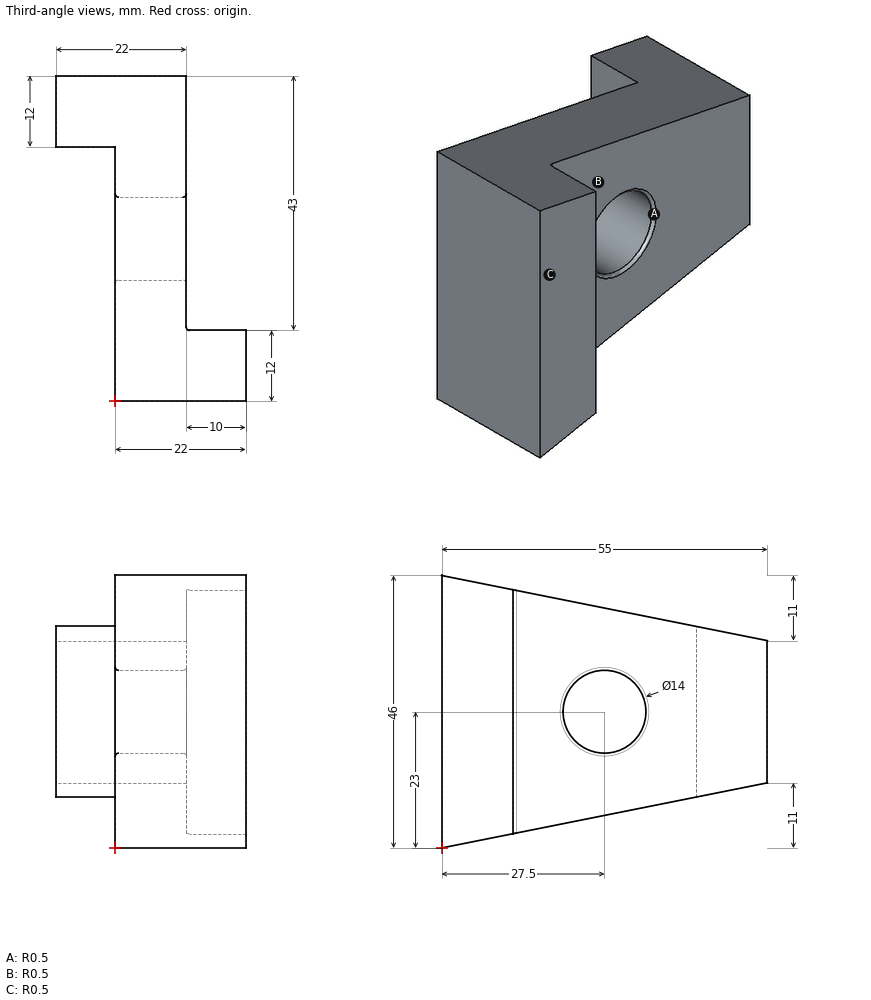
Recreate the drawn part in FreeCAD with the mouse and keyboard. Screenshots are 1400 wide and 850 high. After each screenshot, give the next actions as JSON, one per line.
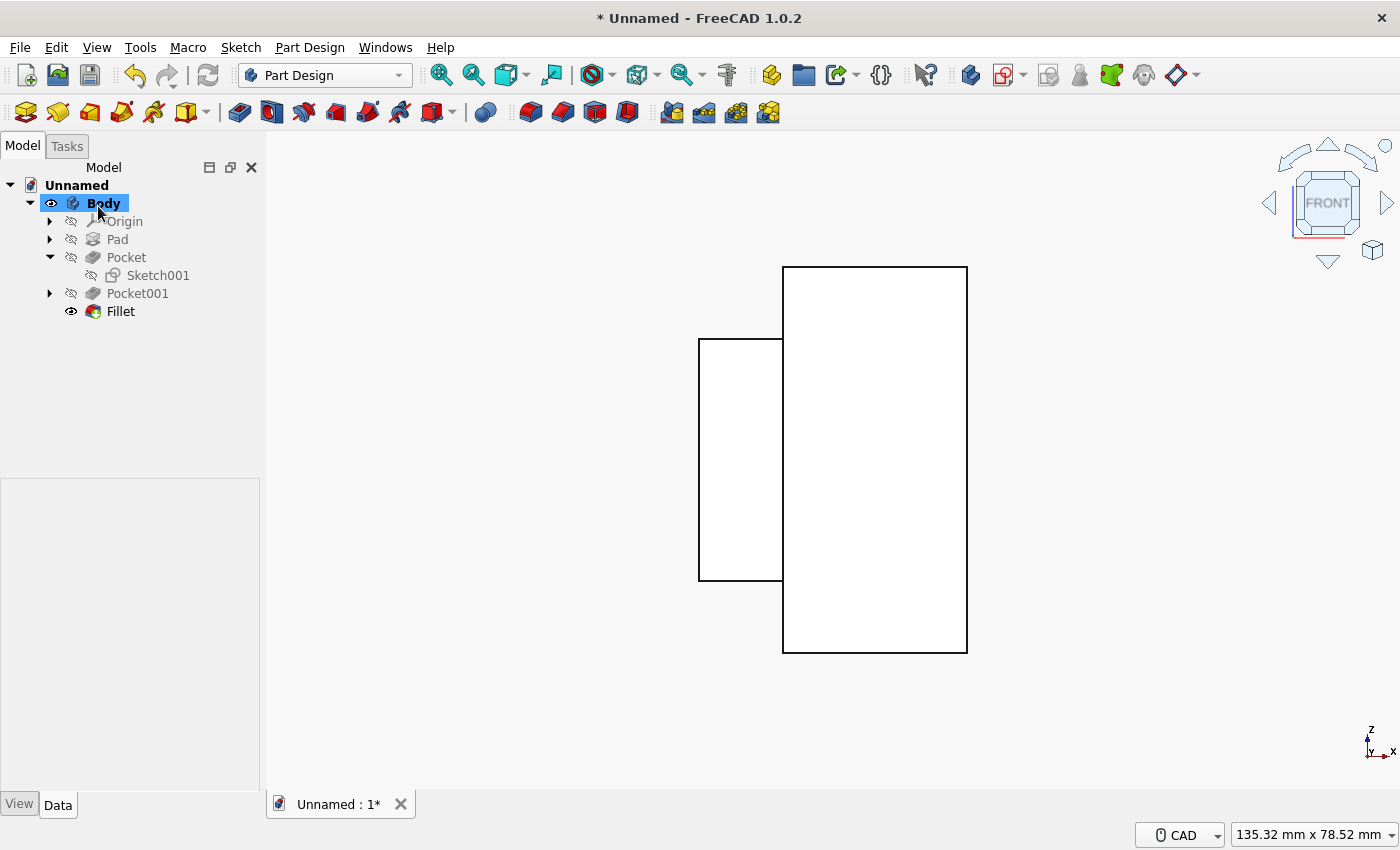
{"action": "key", "text": "3"}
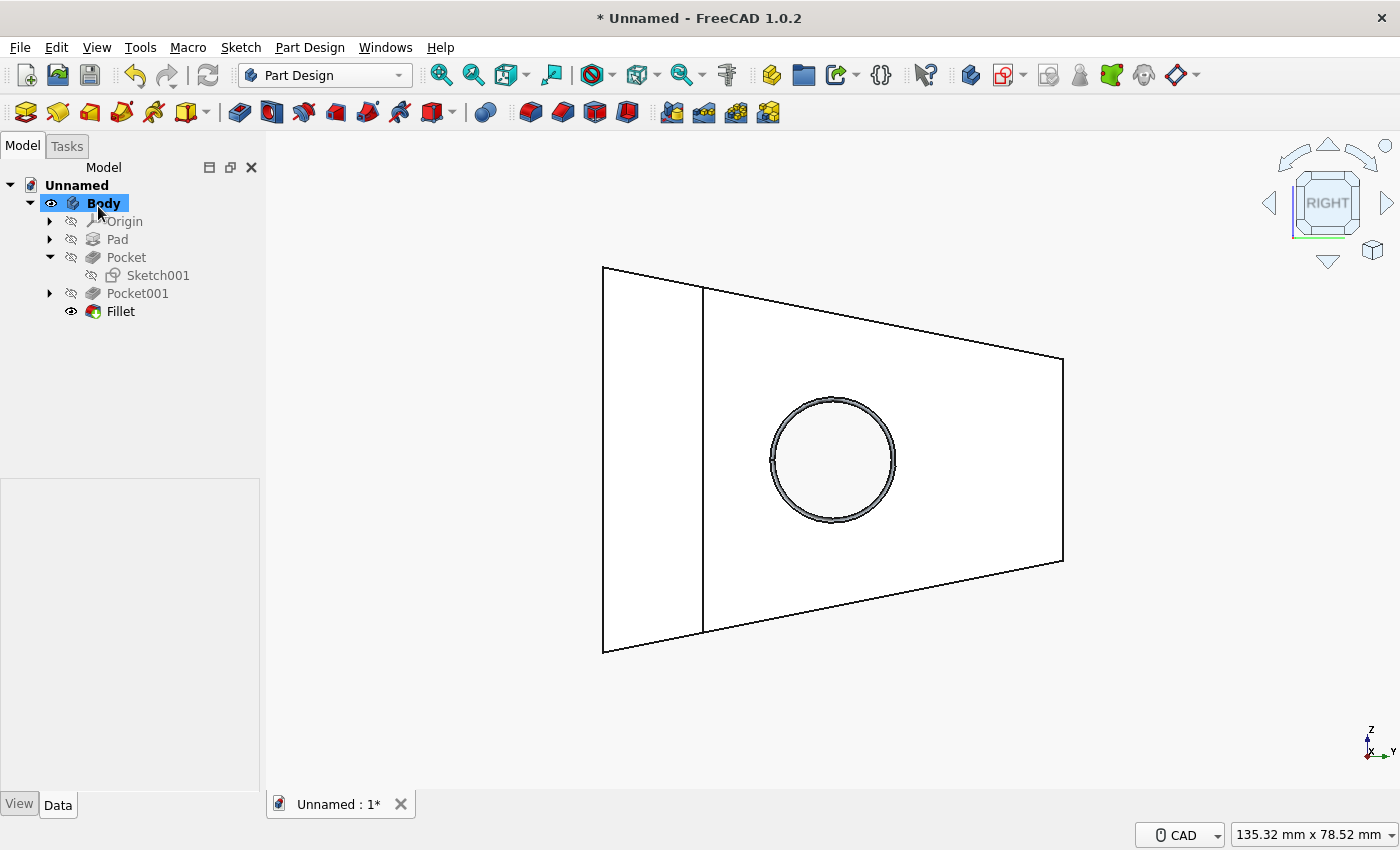
{"action": "key", "text": "5"}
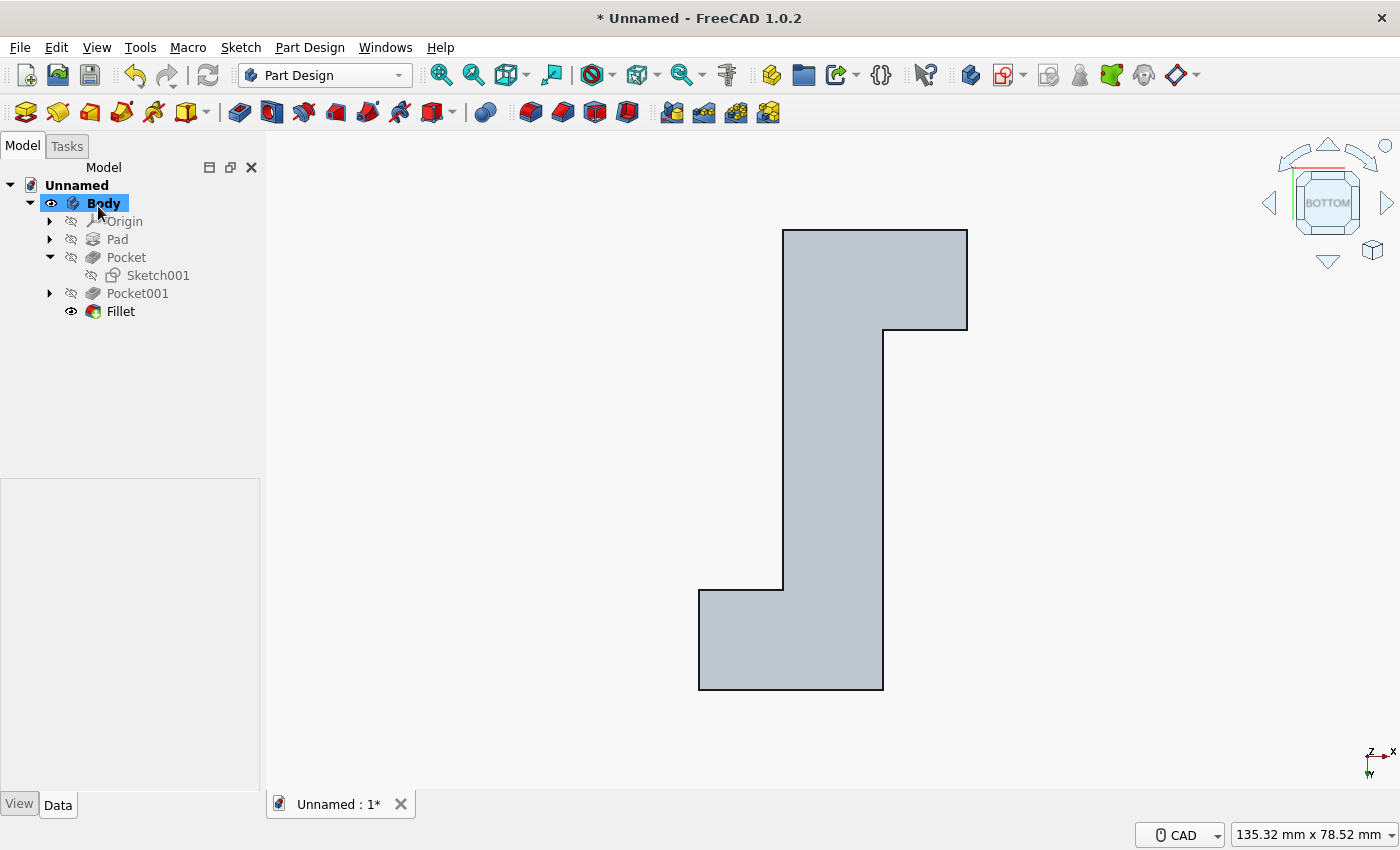
{"action": "key", "text": "4"}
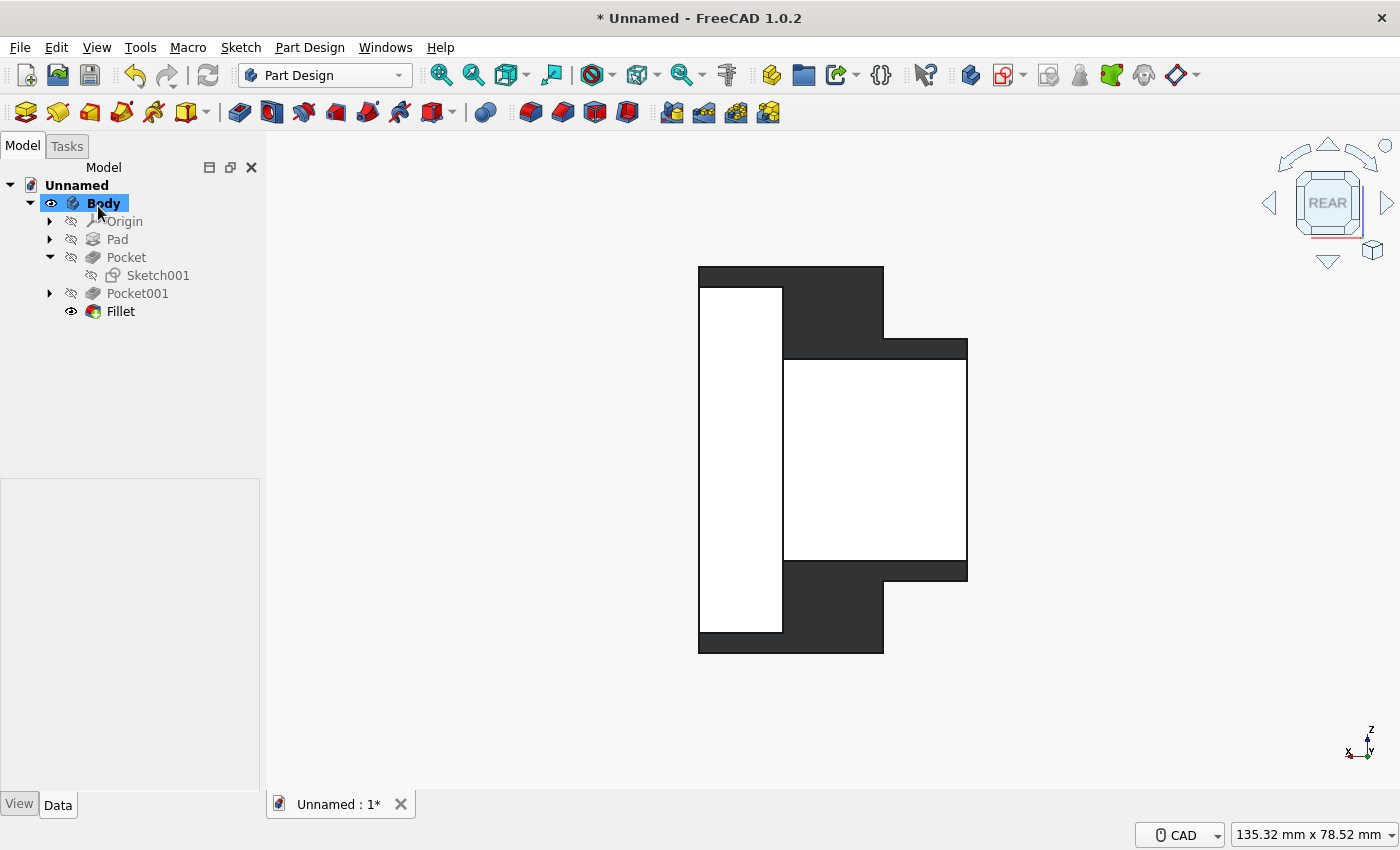
{"action": "key", "text": "6"}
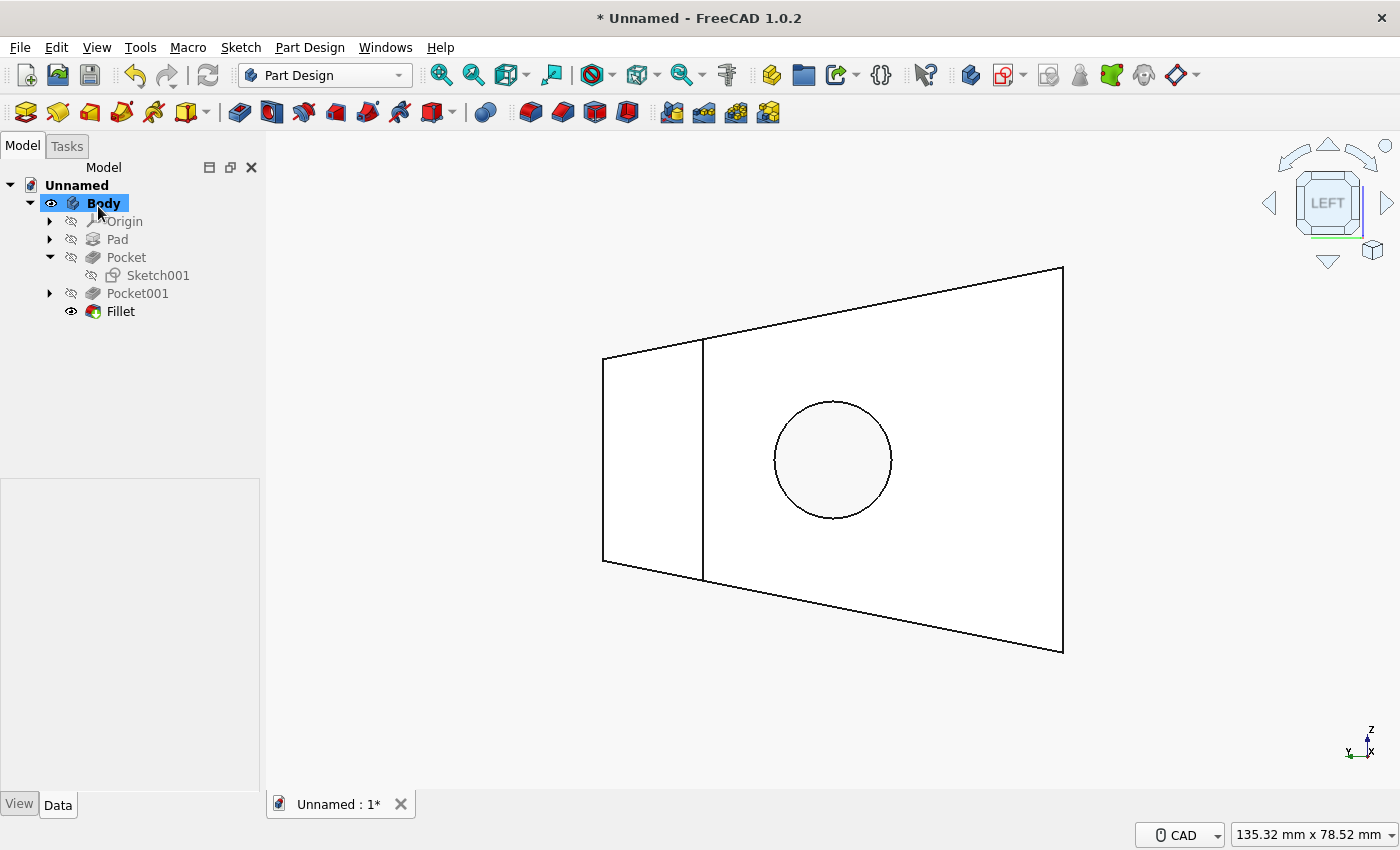
{"action": "left_click", "coordinate": [774, 459]}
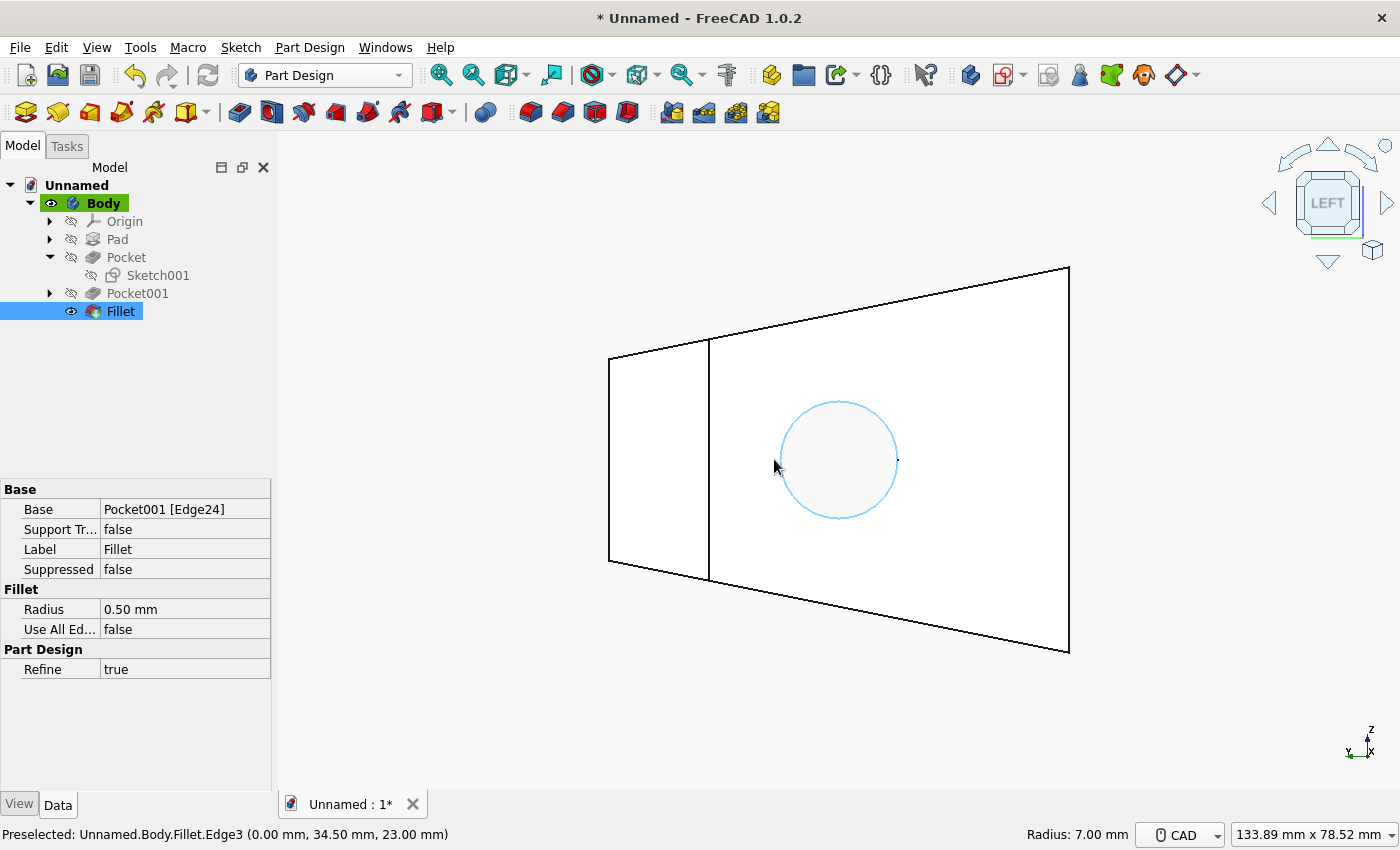
{"action": "left_click", "coordinate": [532, 112]}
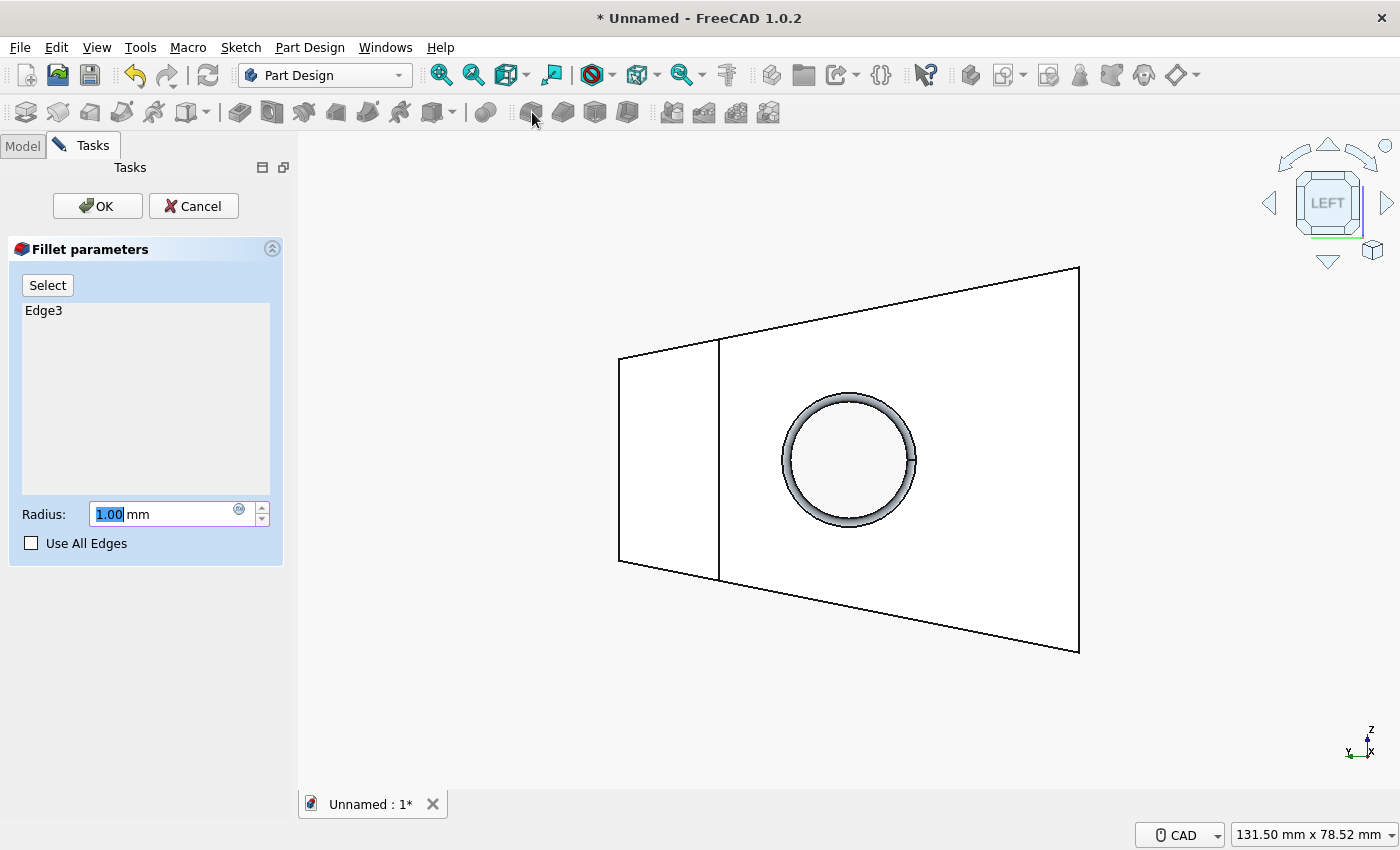
{"action": "type", "text": "0.5"}
{"action": "key", "text": "Tab"}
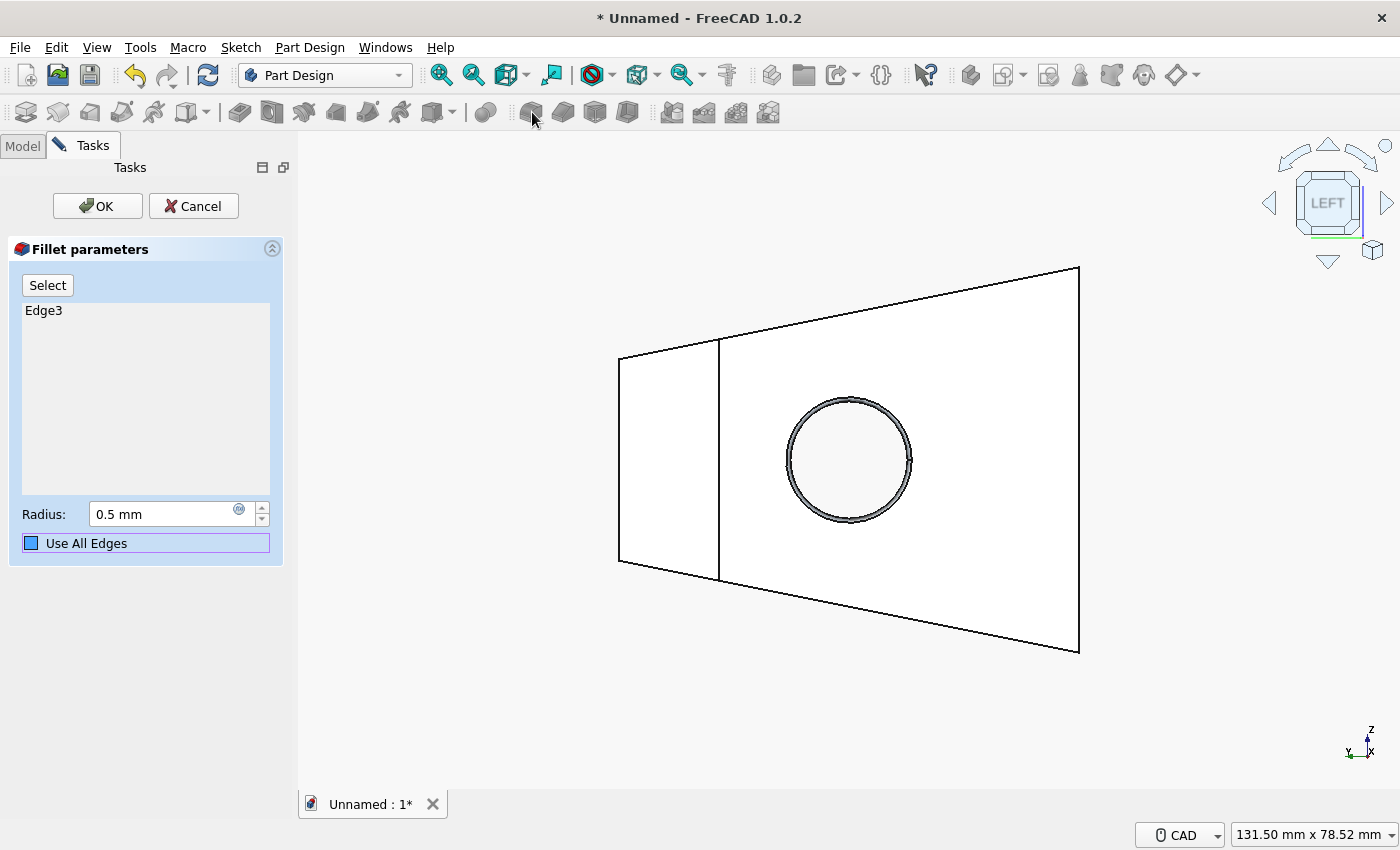
{"action": "left_click", "coordinate": [98, 206]}